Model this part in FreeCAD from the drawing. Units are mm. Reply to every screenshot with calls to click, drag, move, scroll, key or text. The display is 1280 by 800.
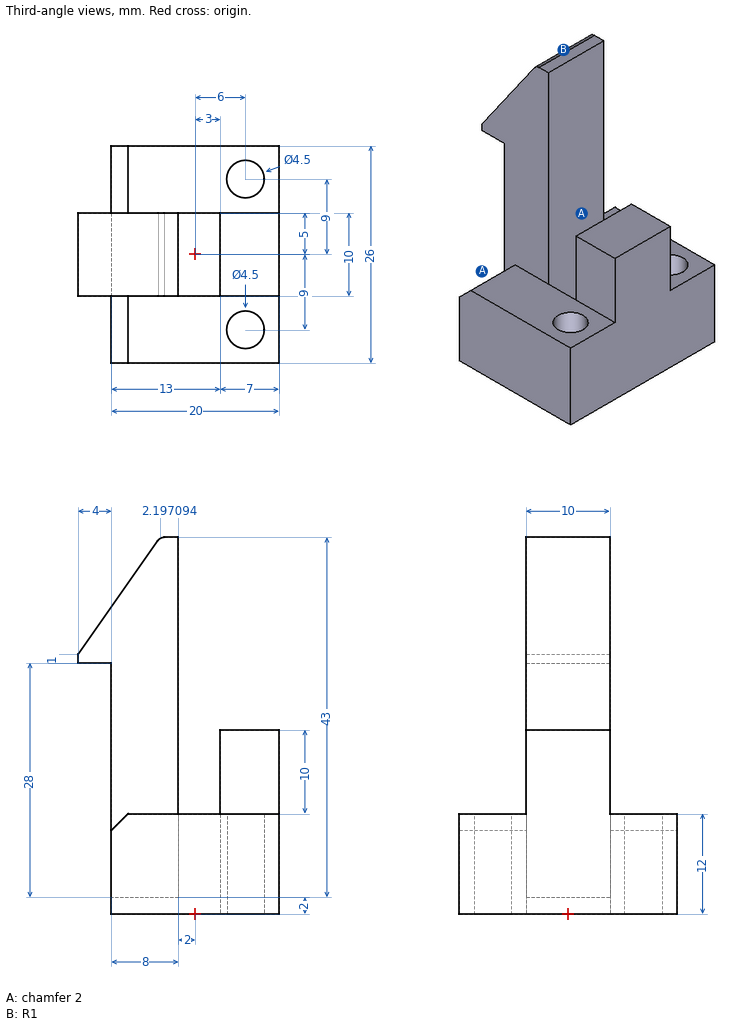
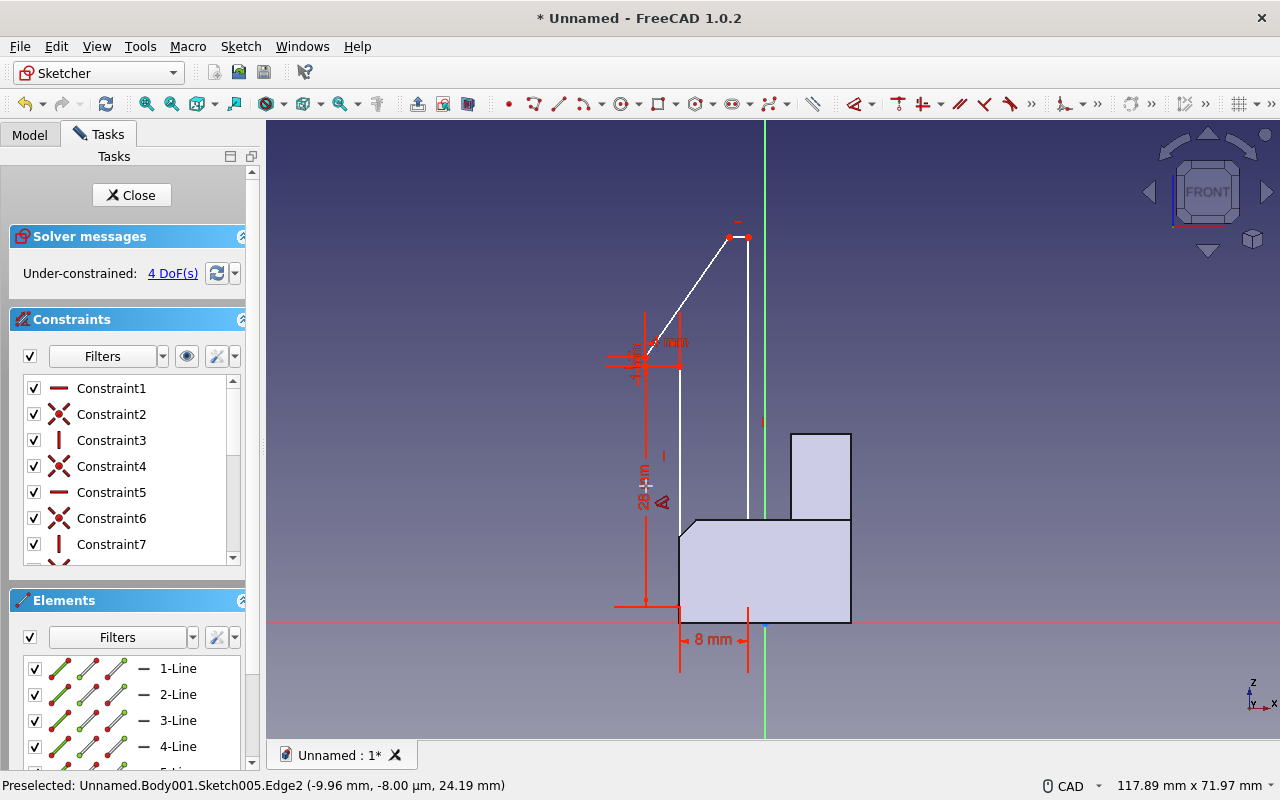
click(748, 348)
click(782, 422)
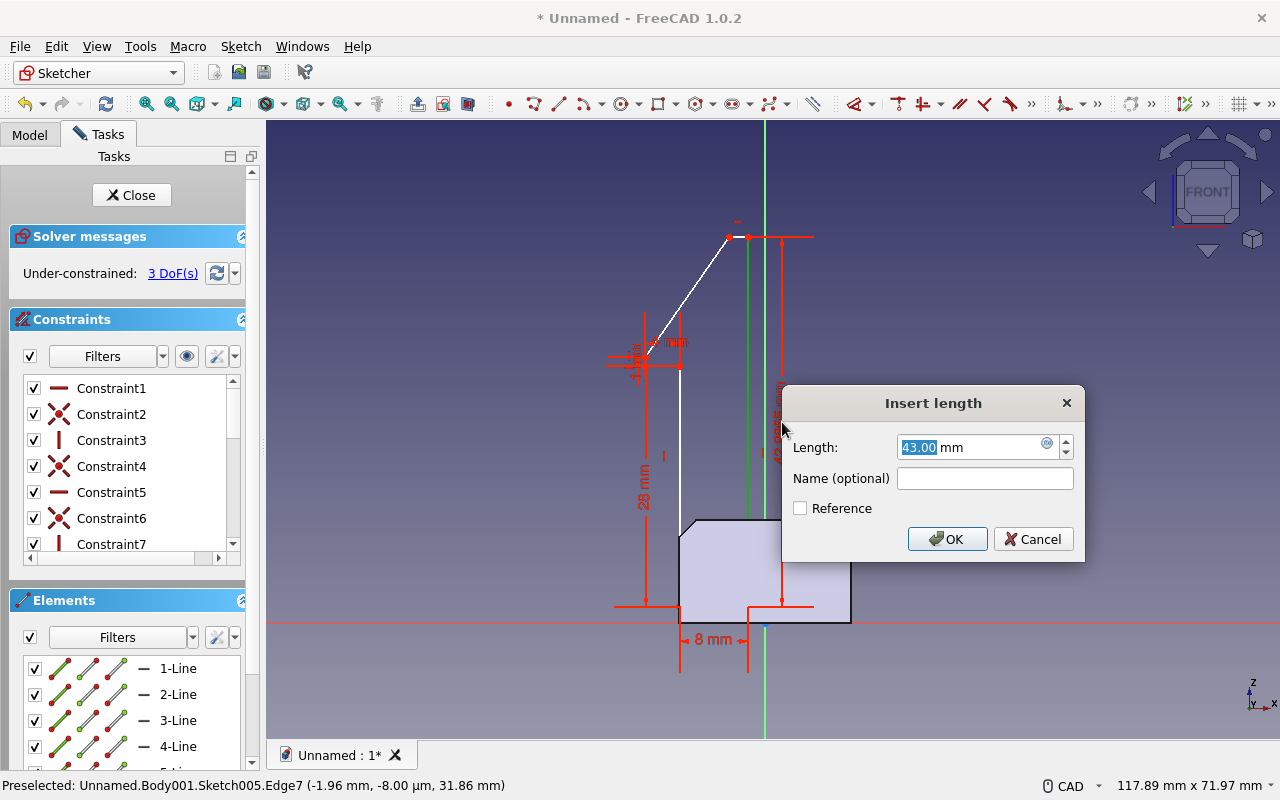
text(43)
key(Return)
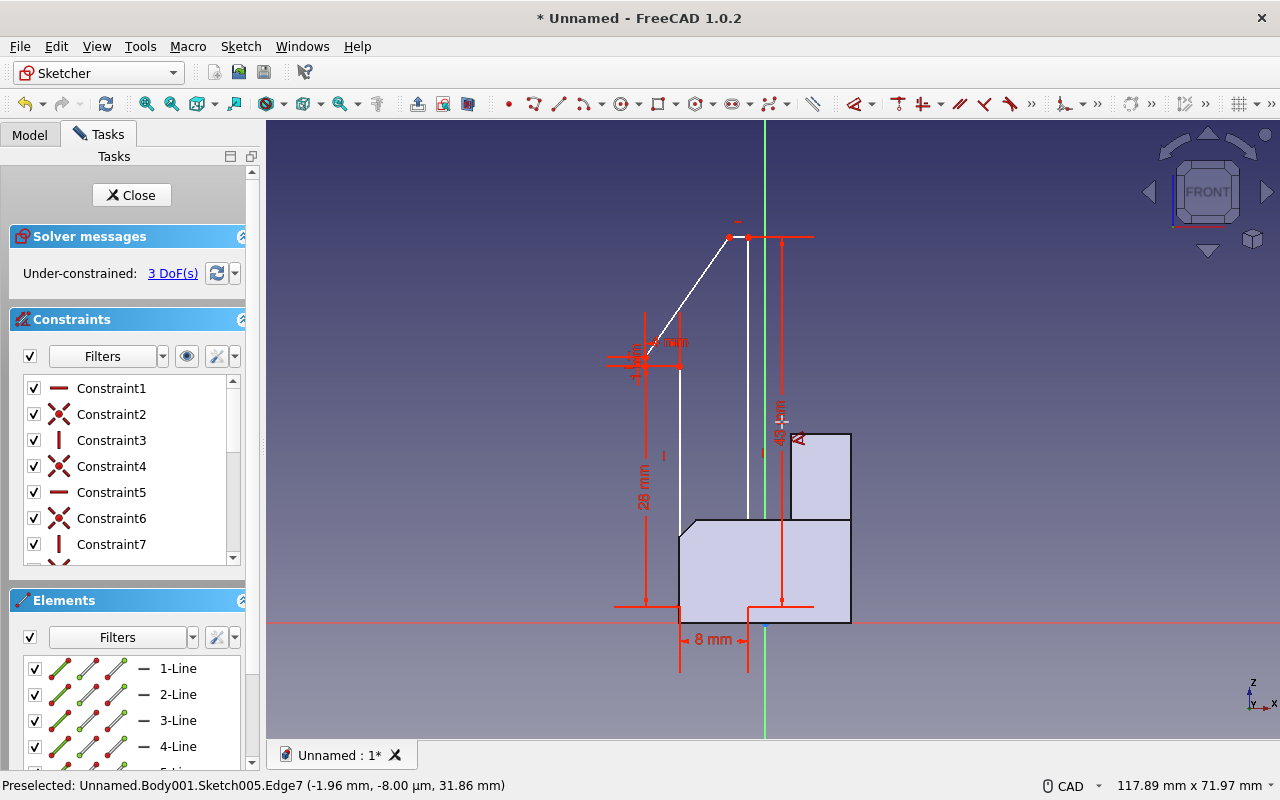
scroll(748, 607, up, 5)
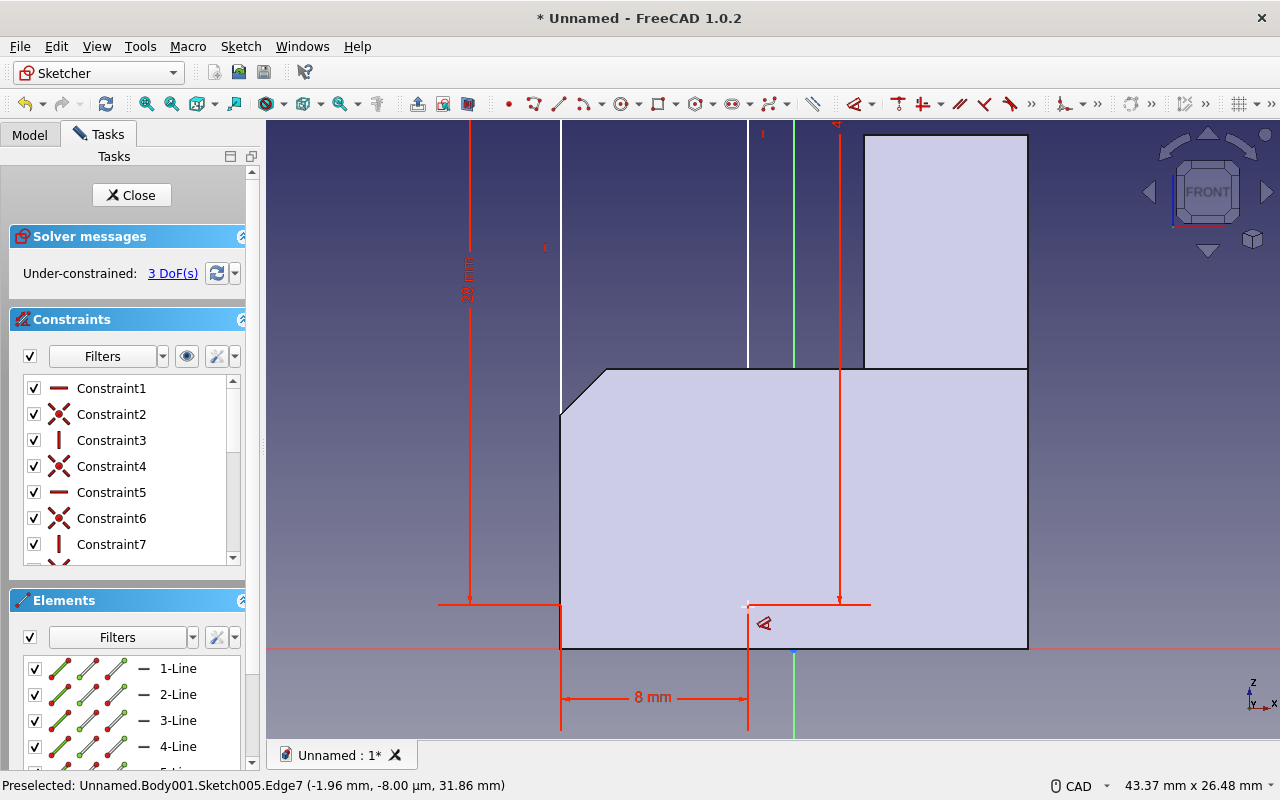
click(748, 605)
click(771, 683)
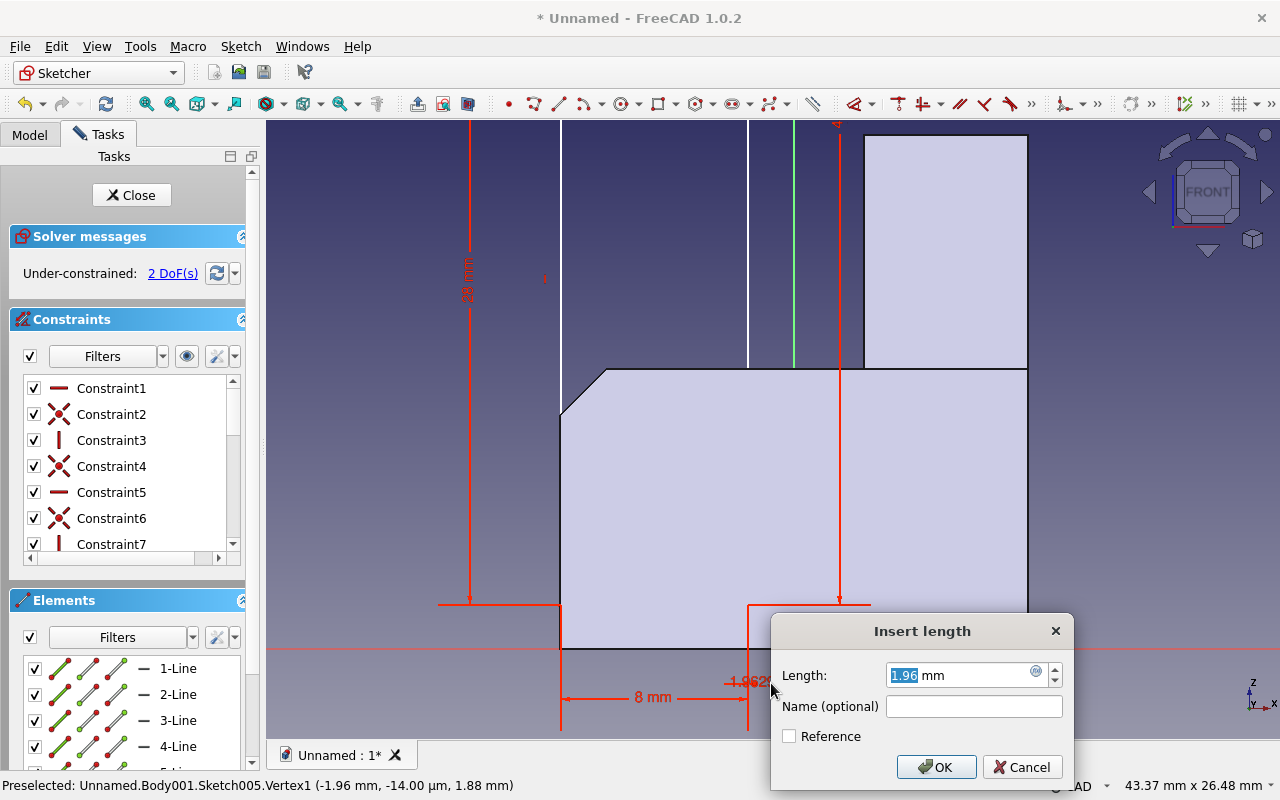
text(2)
key(Return)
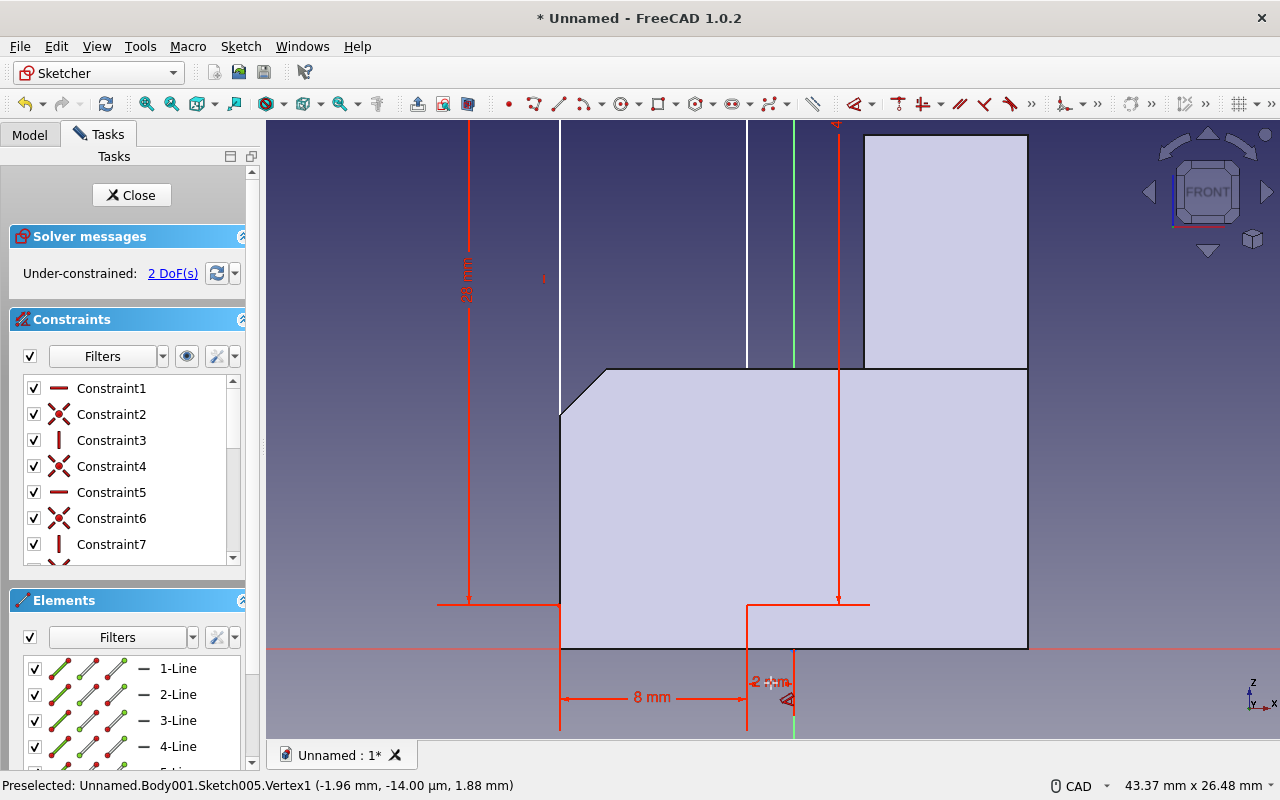
click(747, 605)
click(828, 627)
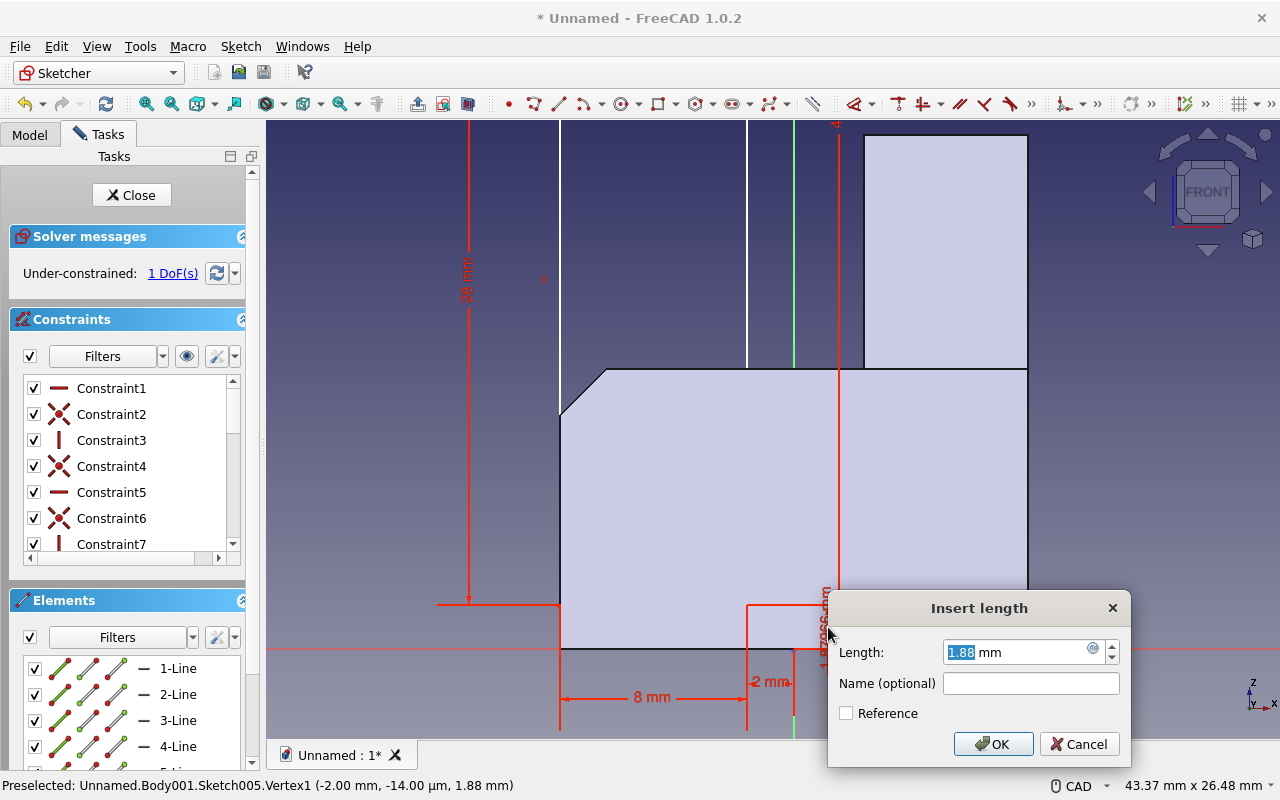
text(2)
key(Return)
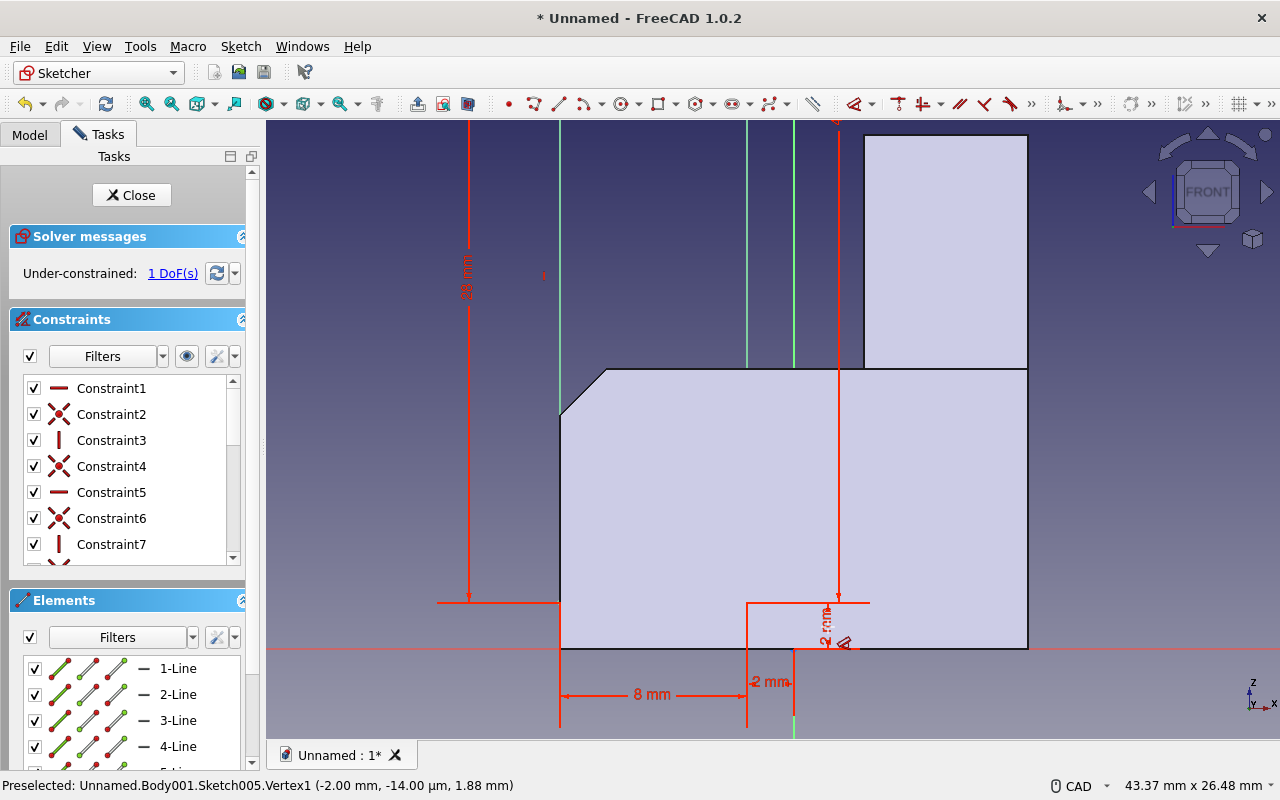
scroll(748, 608, down, 5)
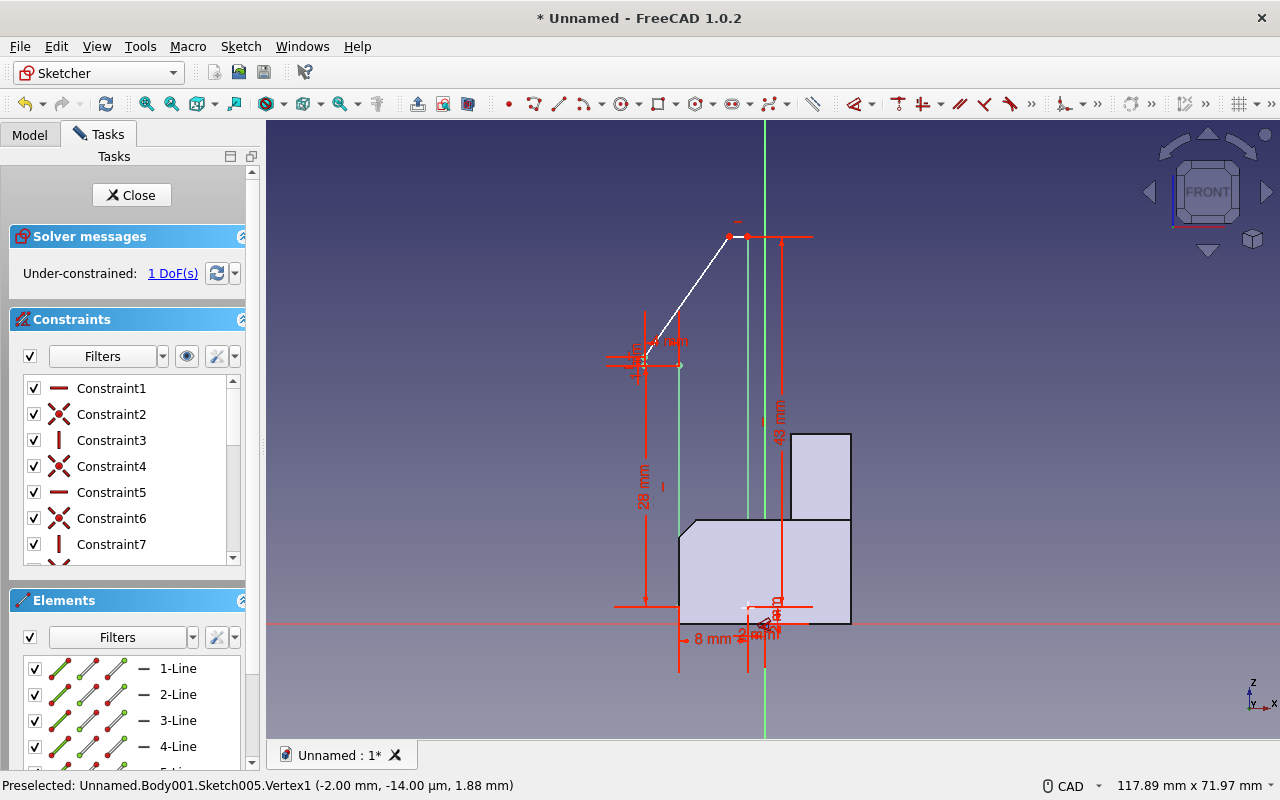
scroll(735, 237, up, 5)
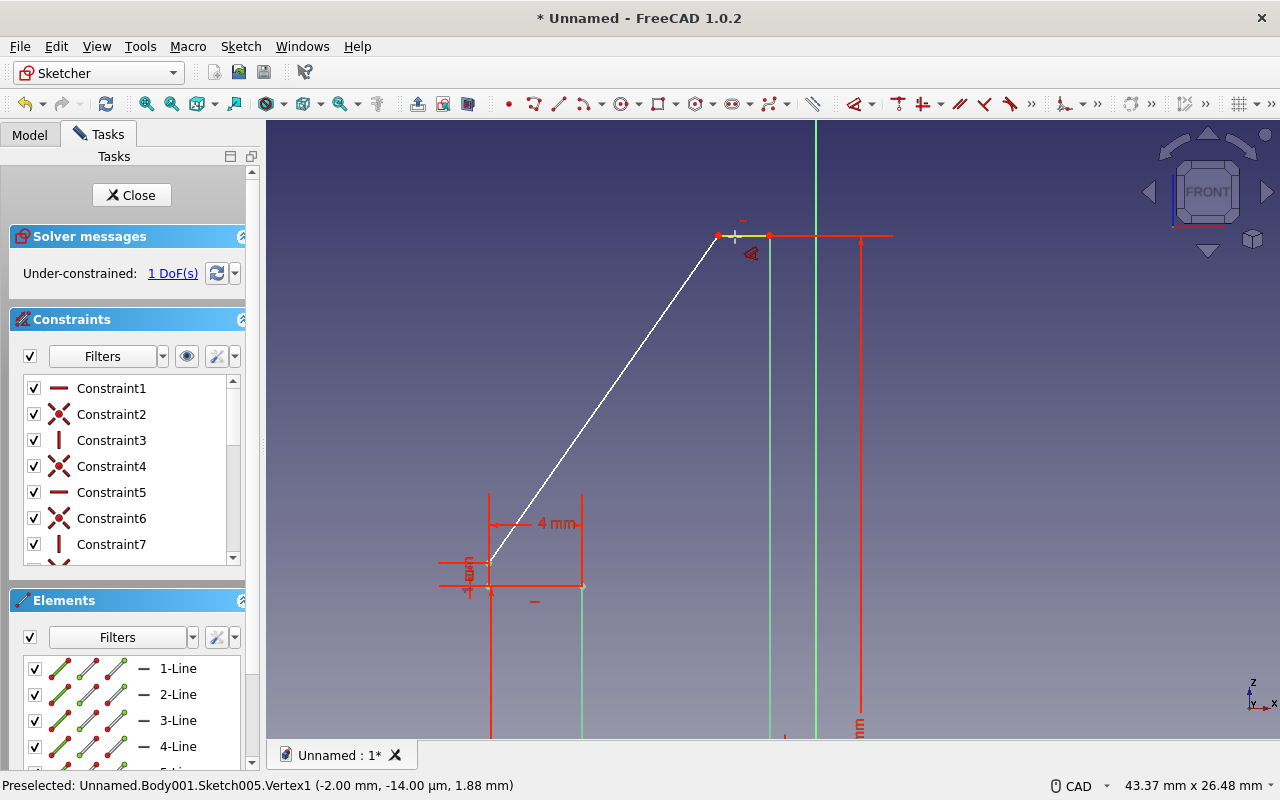
click(734, 236)
click(744, 202)